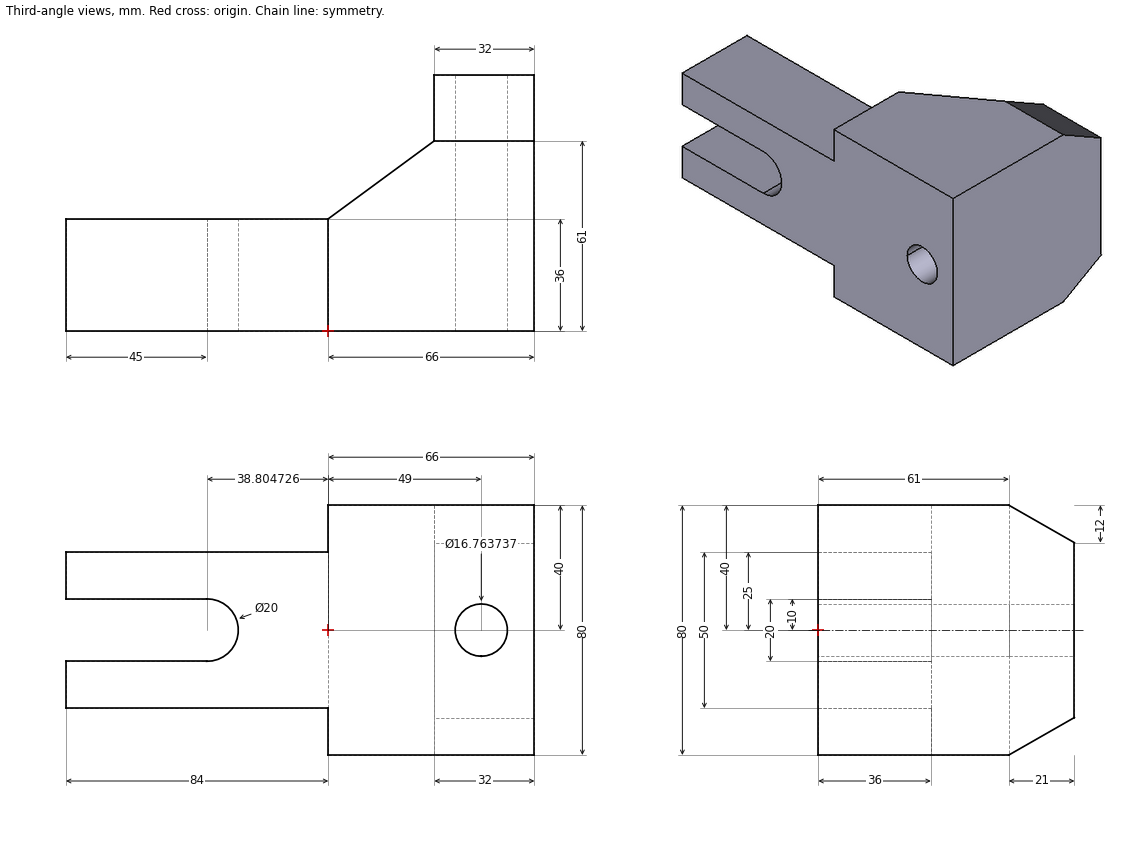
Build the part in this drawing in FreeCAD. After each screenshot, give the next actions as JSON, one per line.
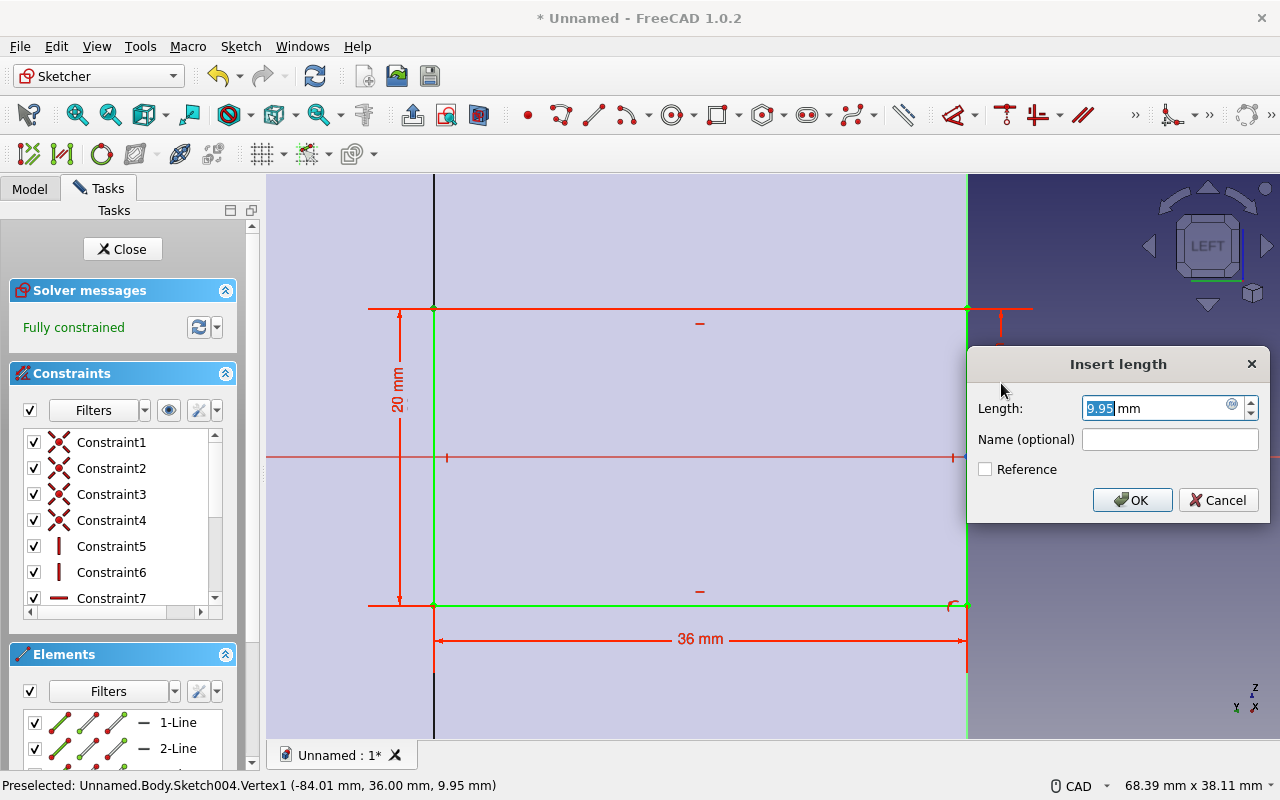
{"action": "type", "text": "10"}
{"action": "key", "text": "Return"}
{"action": "key", "text": "Escape"}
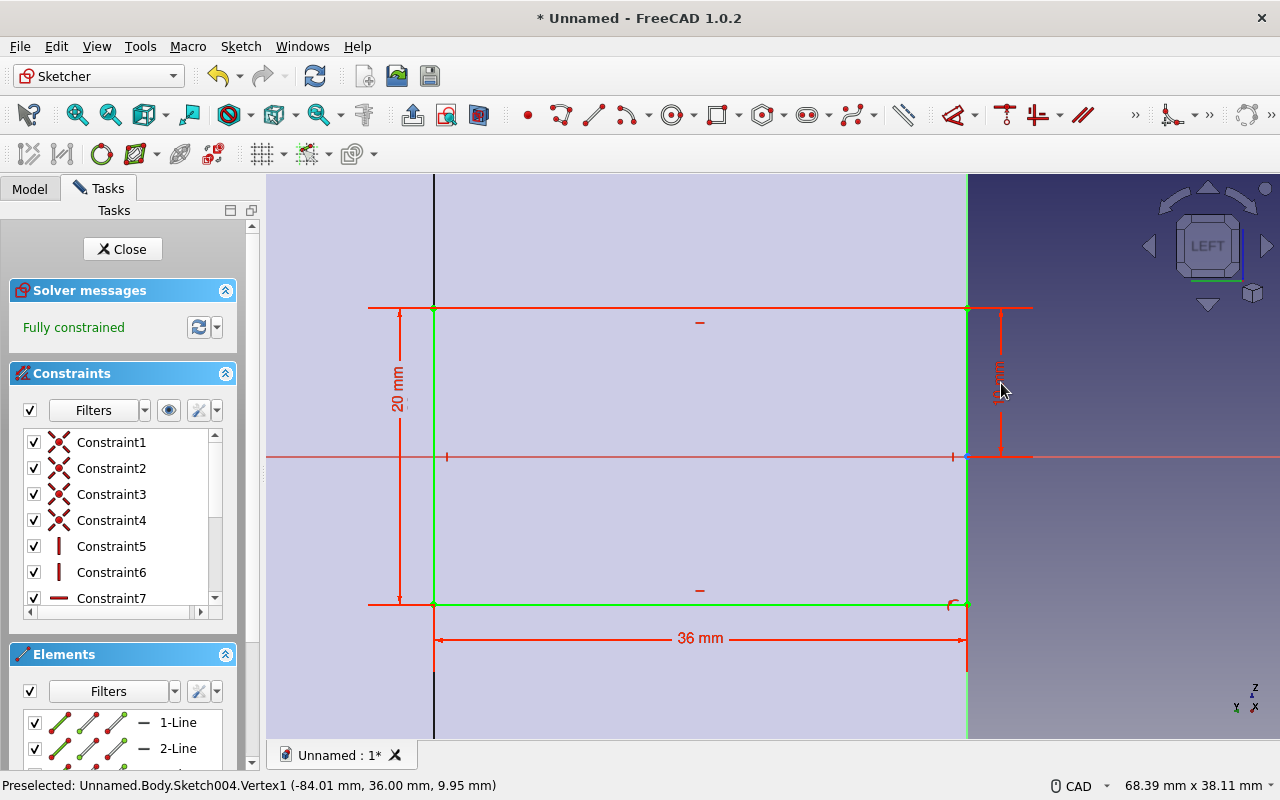
{"action": "left_click", "coordinate": [123, 249]}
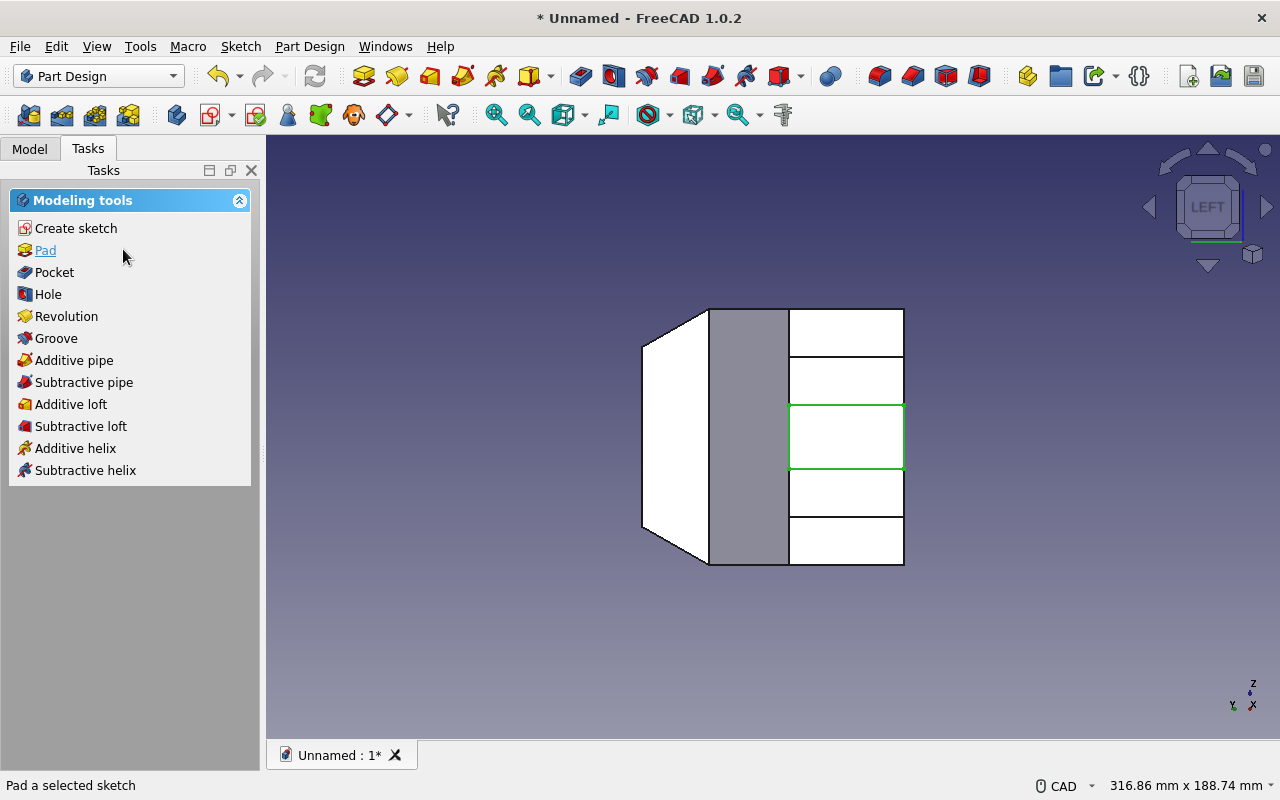
{"action": "left_click", "coordinate": [581, 76]}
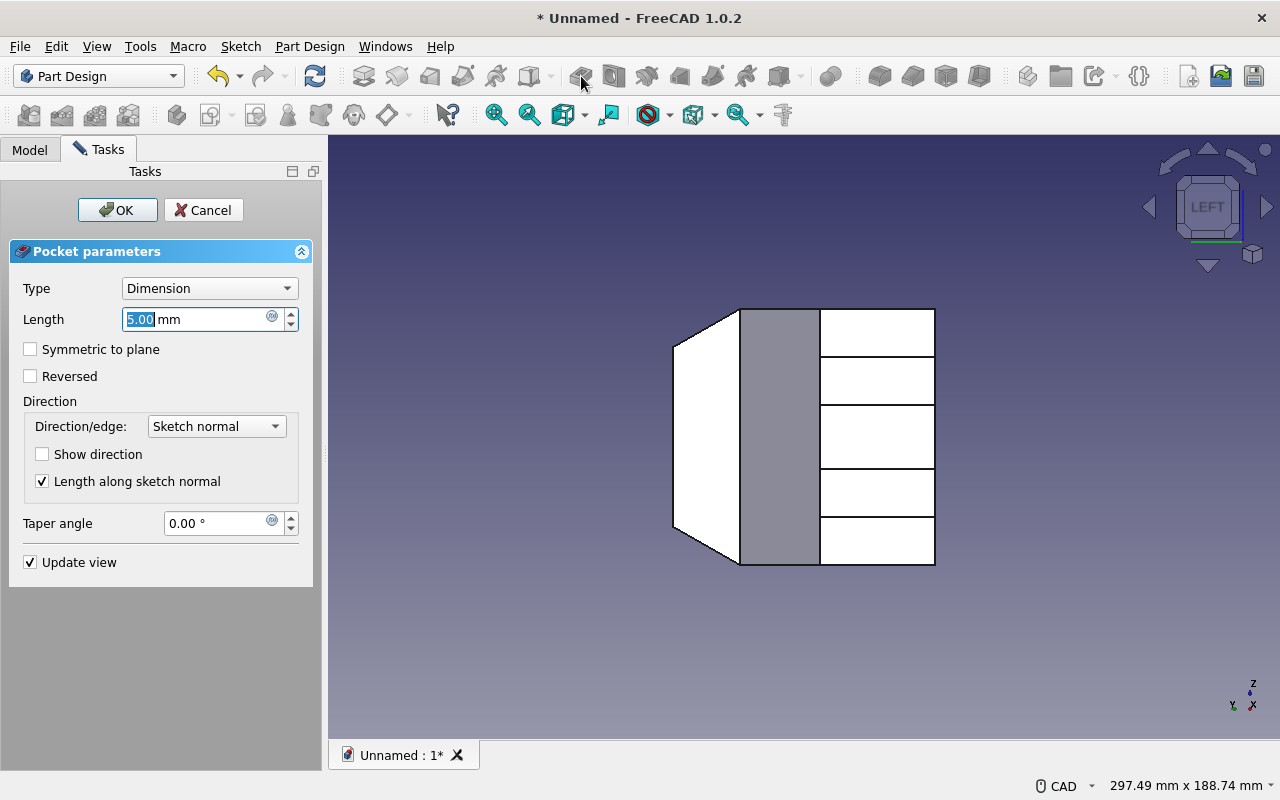
{"action": "type", "text": "45"}
{"action": "key", "text": "Tab"}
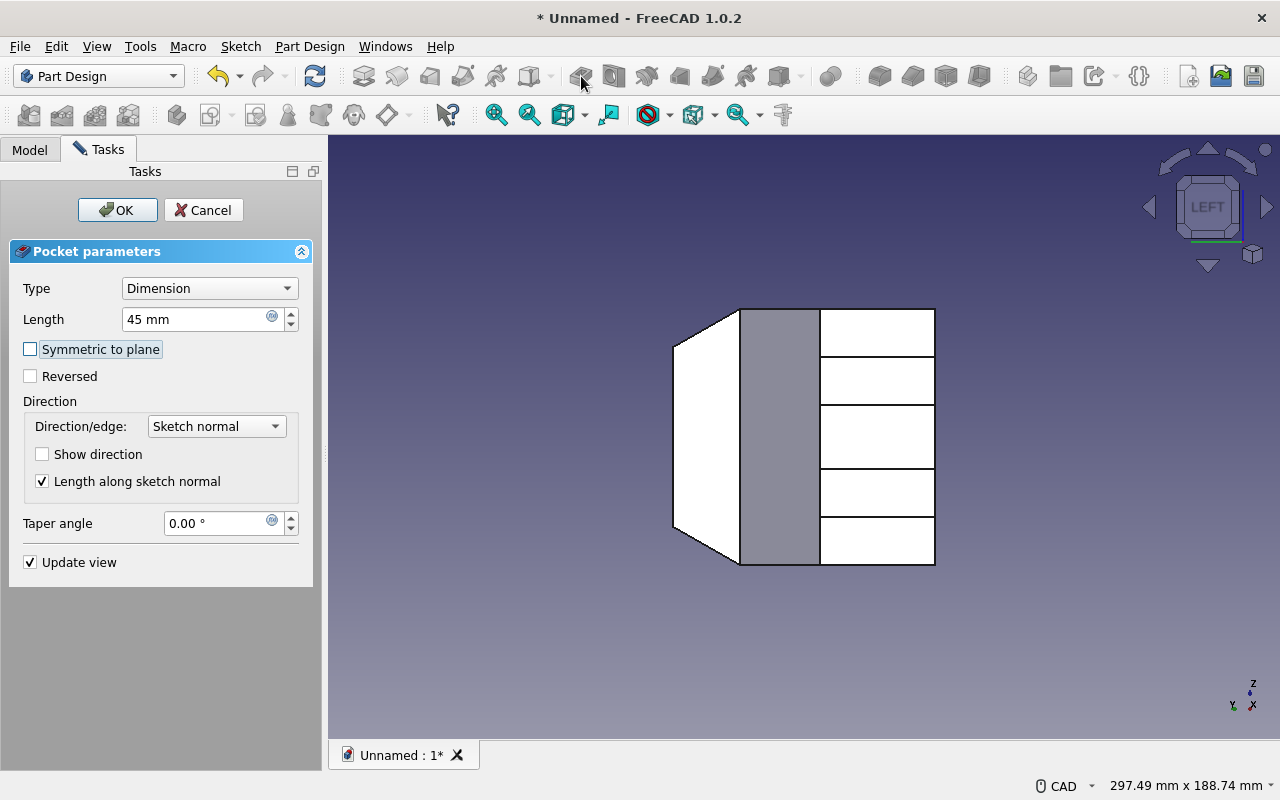
{"action": "left_click", "coordinate": [118, 210]}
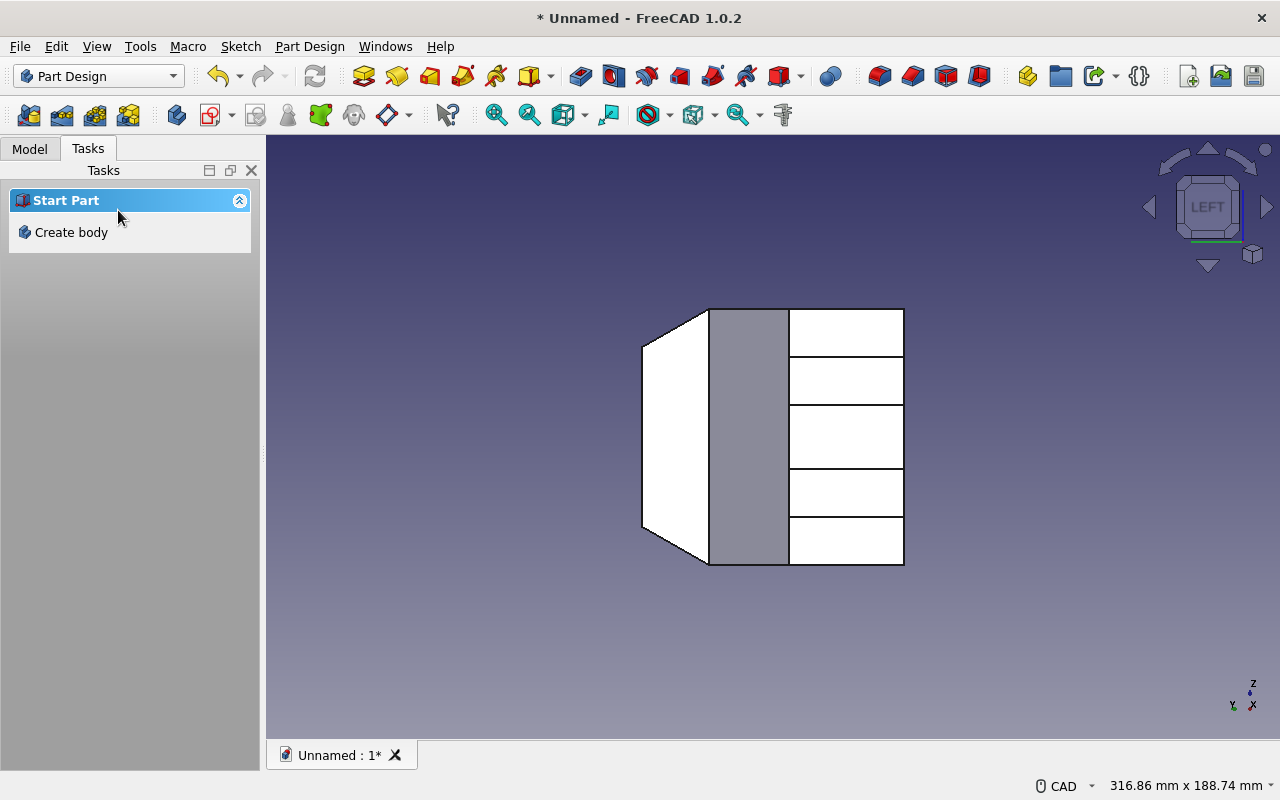
{"action": "key", "text": "v f"}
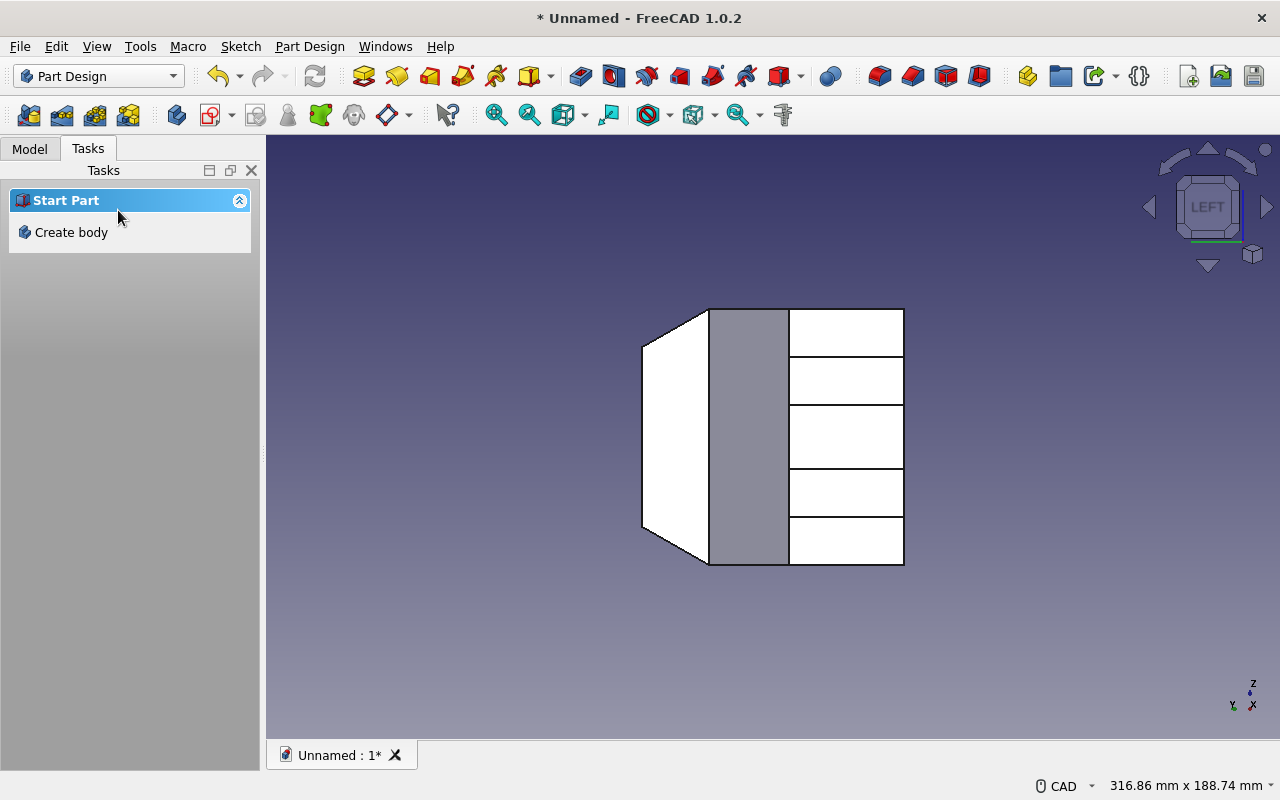
{"action": "key", "text": "4"}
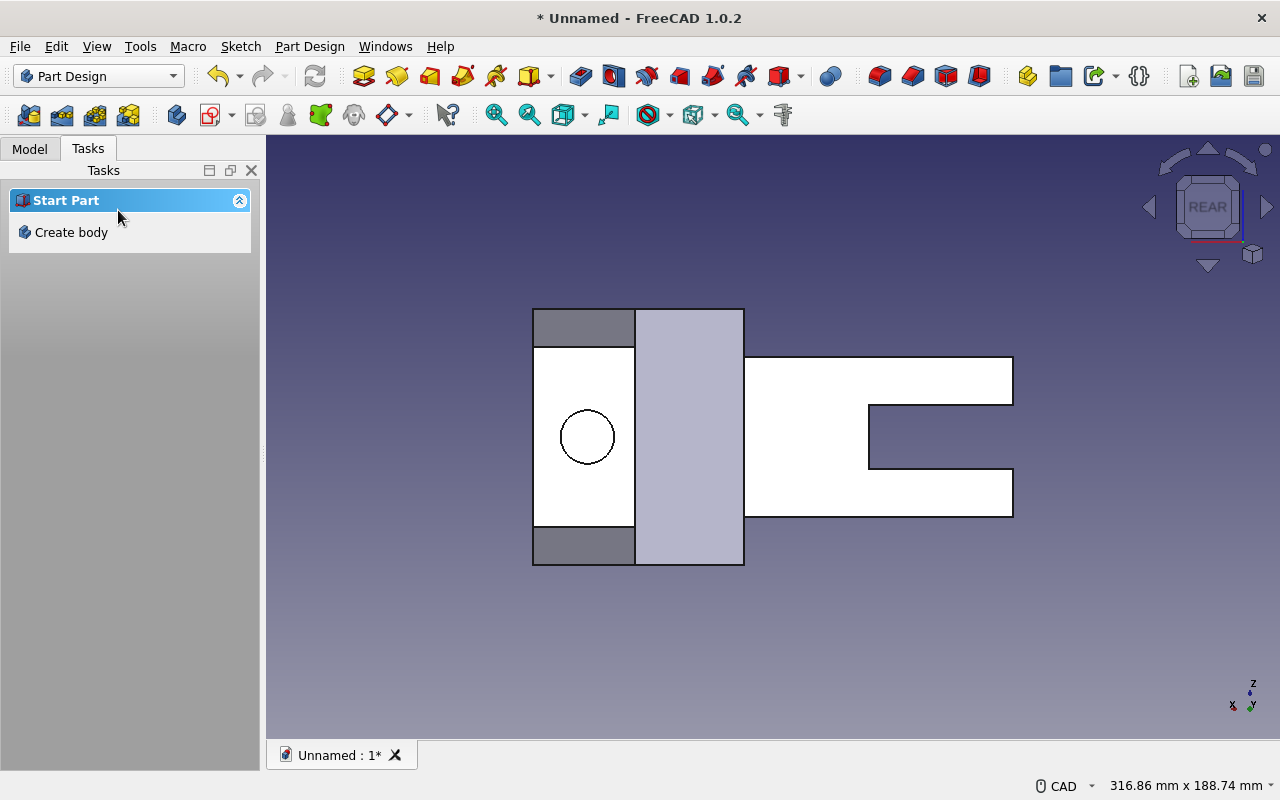
{"action": "left_click", "coordinate": [802, 436]}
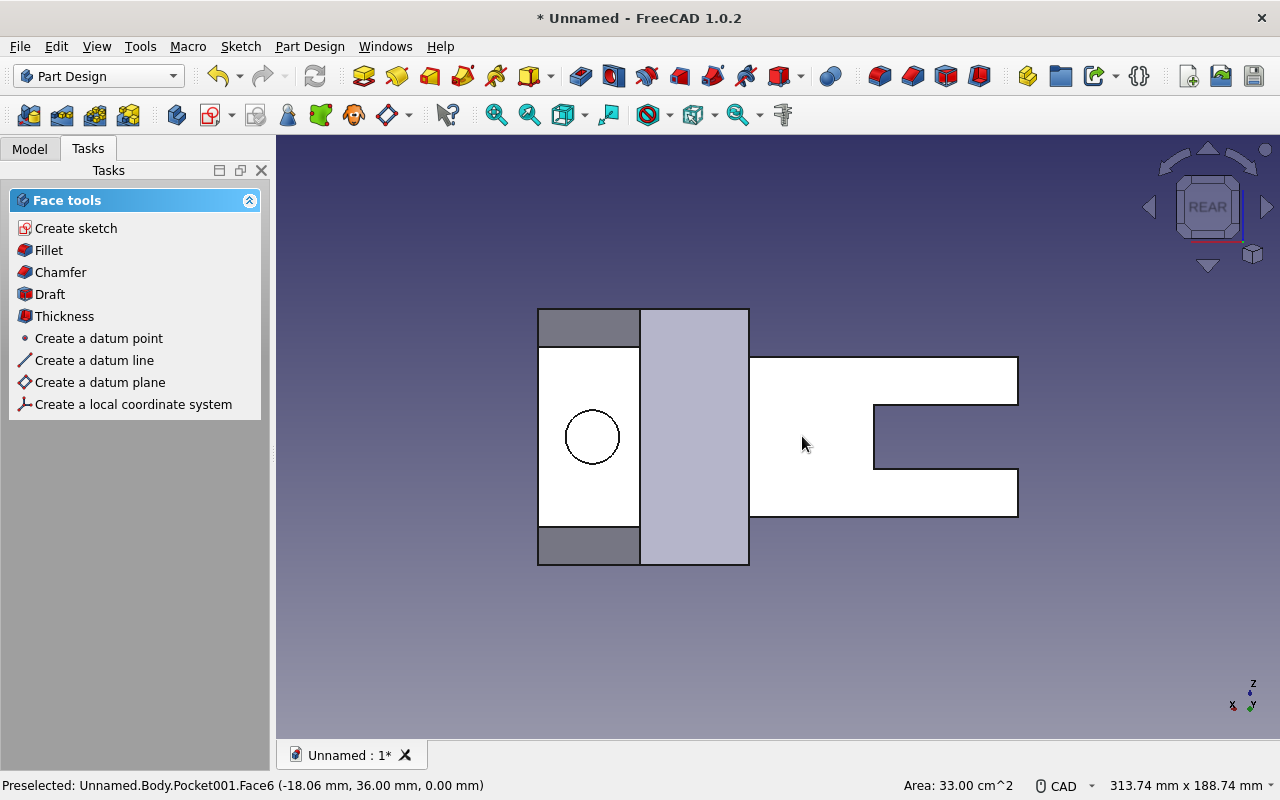
{"action": "left_click", "coordinate": [210, 116]}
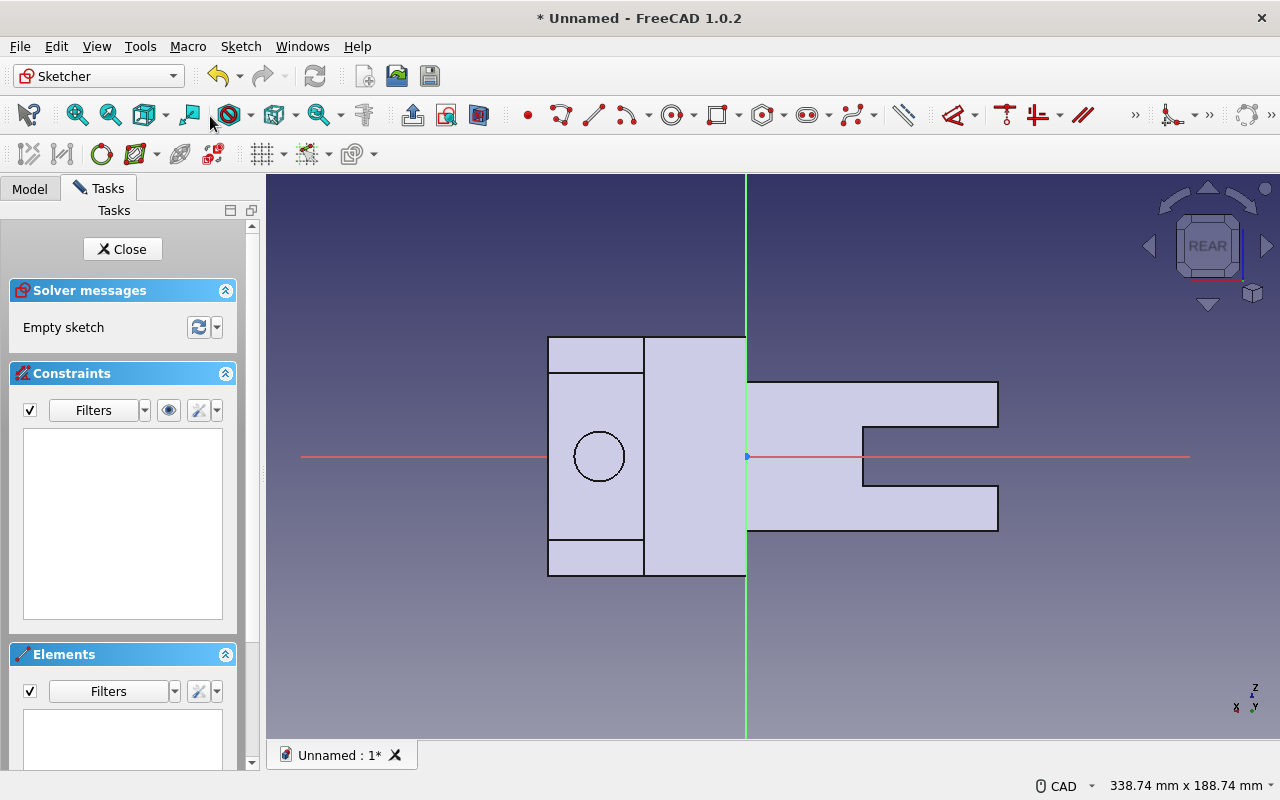
{"action": "scroll", "coordinate": [857, 456], "scroll_direction": "up", "scroll_amount": 7}